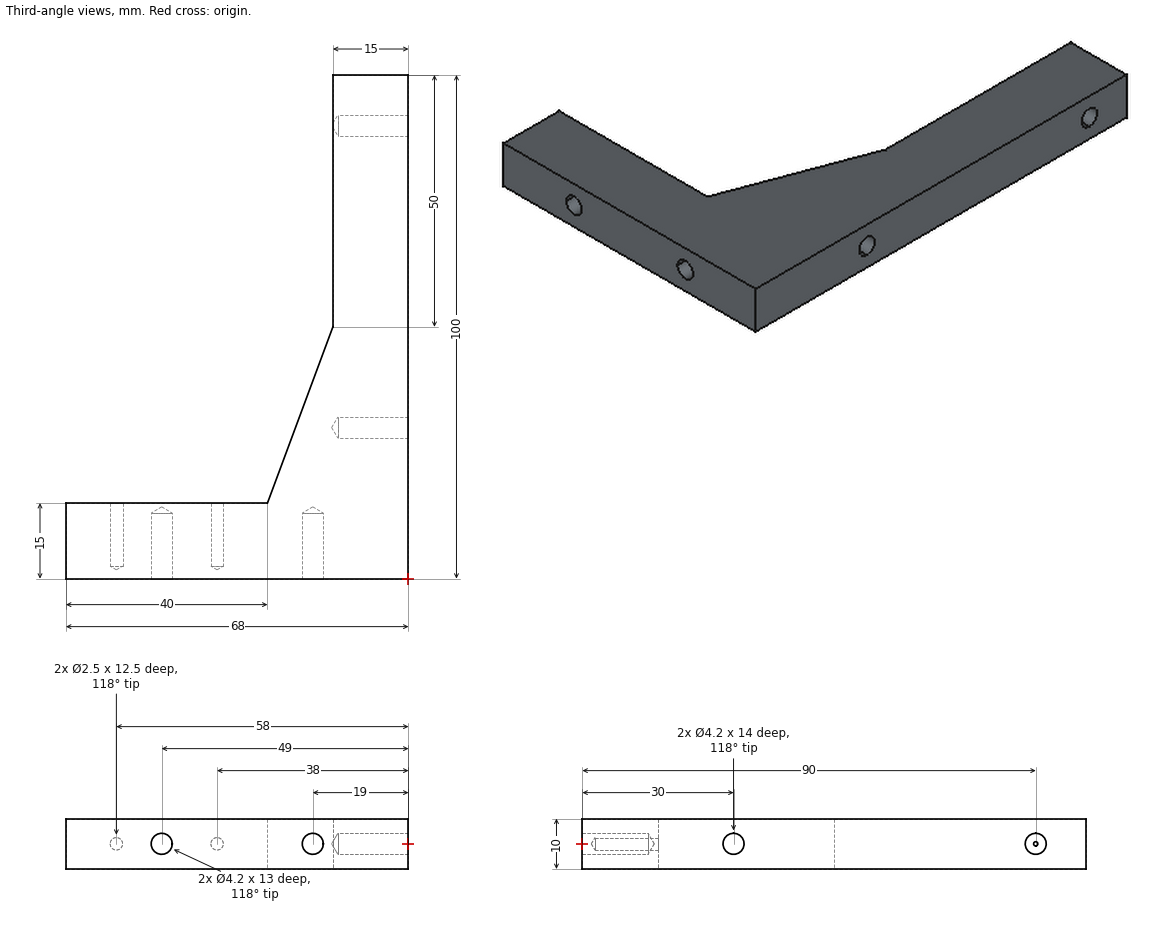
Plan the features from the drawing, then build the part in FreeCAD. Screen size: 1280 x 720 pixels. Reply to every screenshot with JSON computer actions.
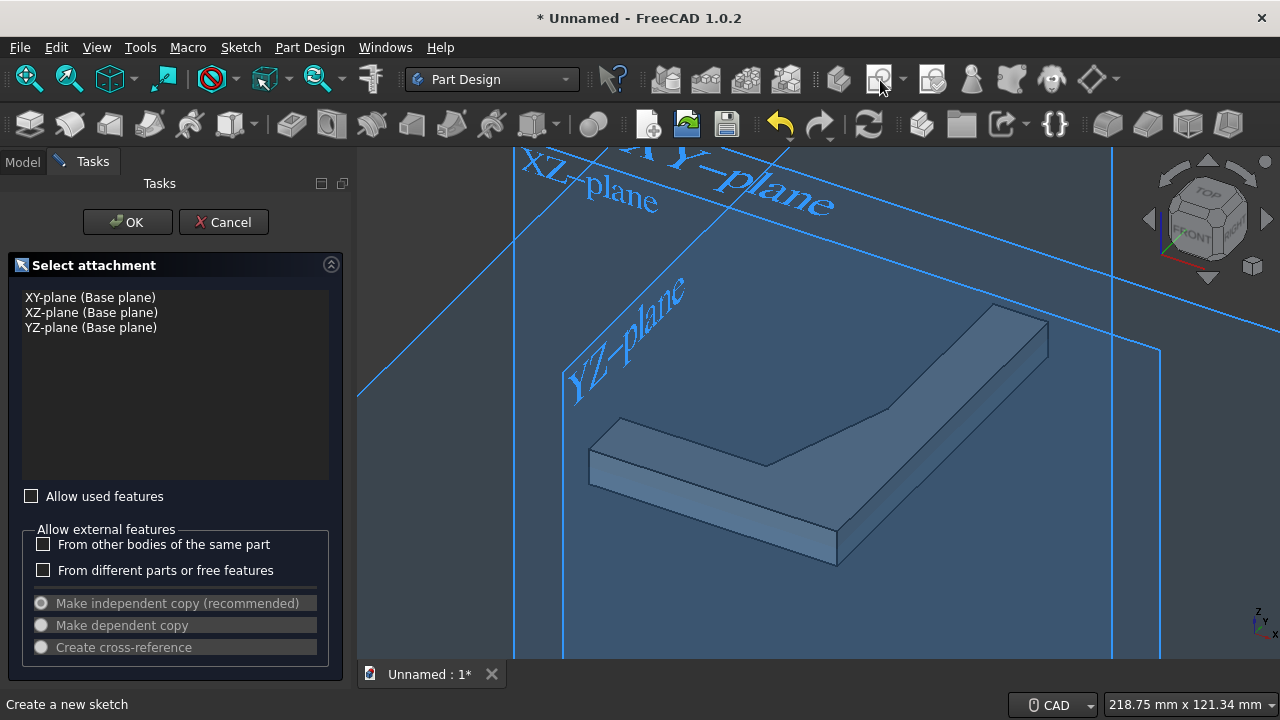
{"action": "left_click", "coordinate": [82, 312]}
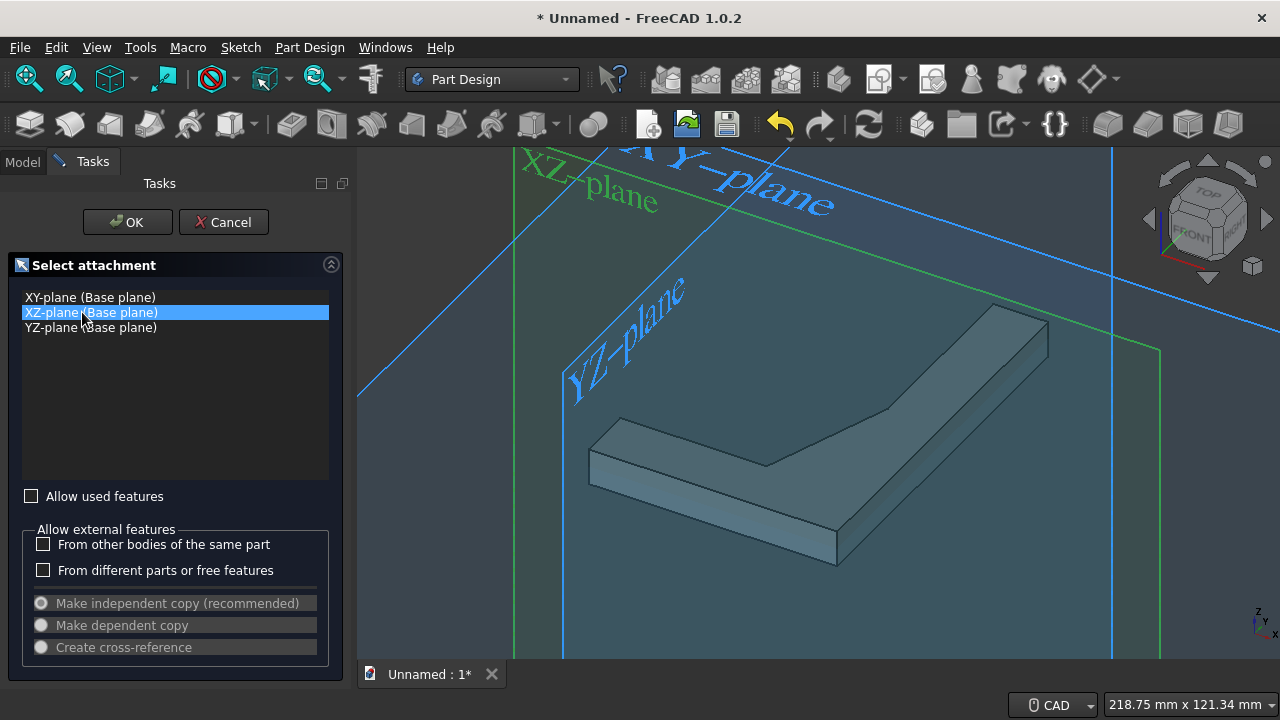
{"action": "left_click", "coordinate": [128, 222]}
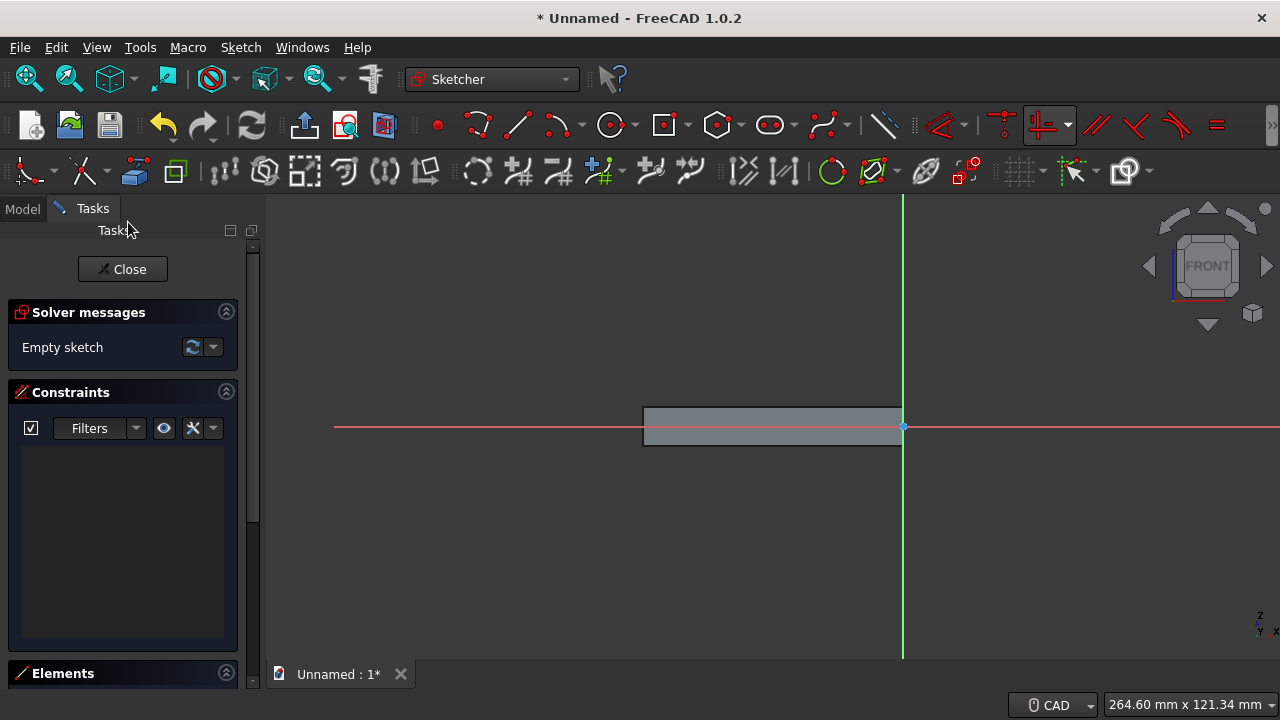
{"action": "scroll", "coordinate": [864, 427], "scroll_direction": "up", "scroll_amount": 5}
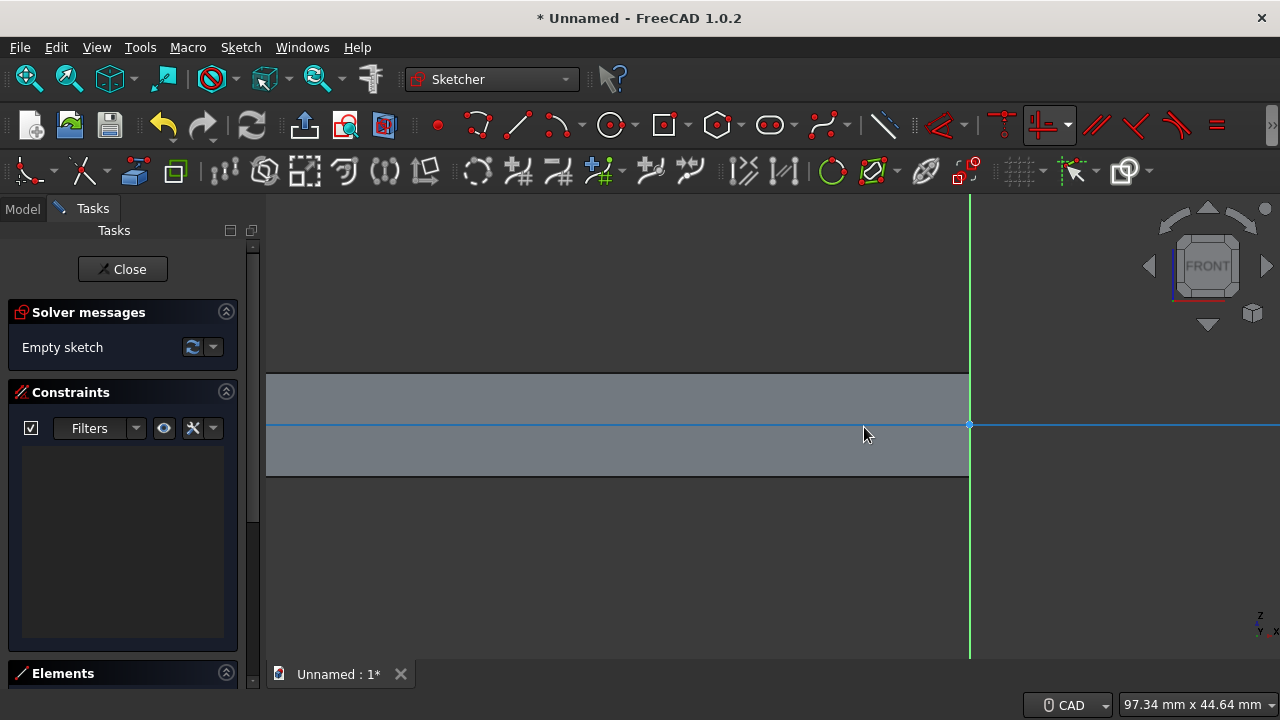
{"action": "key", "text": "g c"}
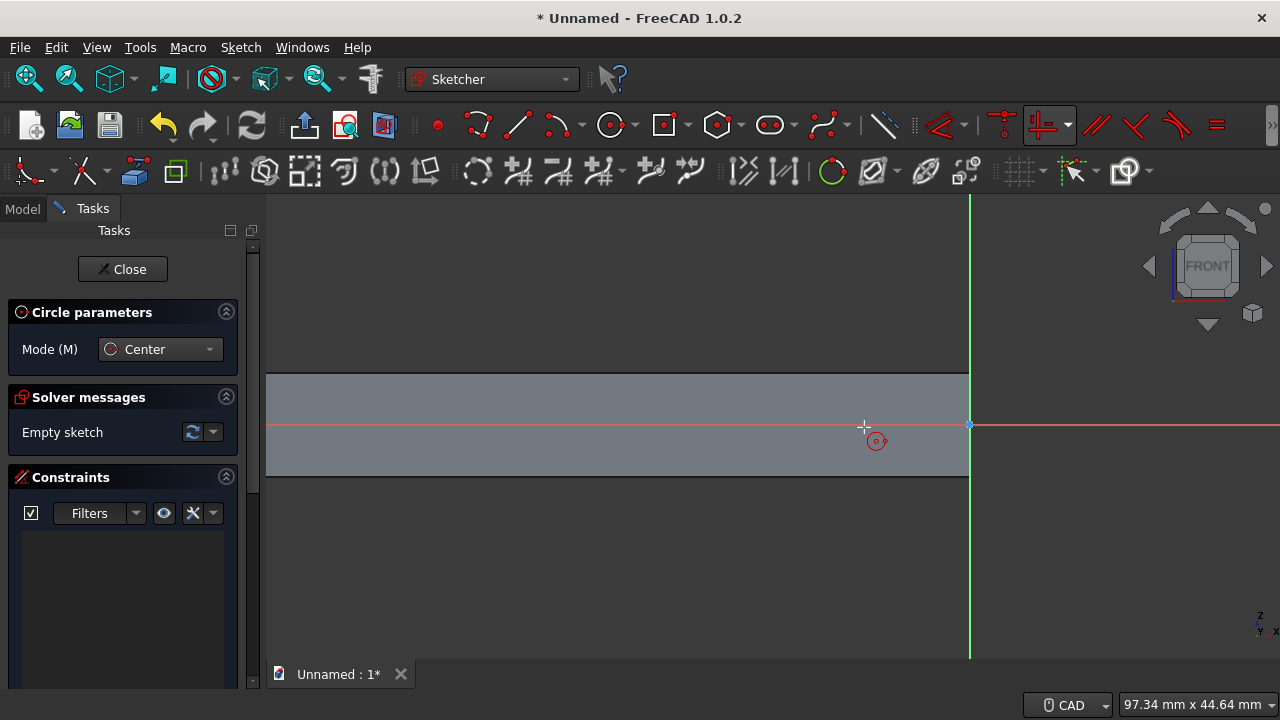
{"action": "left_click", "coordinate": [459, 425]}
{"action": "mouse_move", "coordinate": [475, 409]}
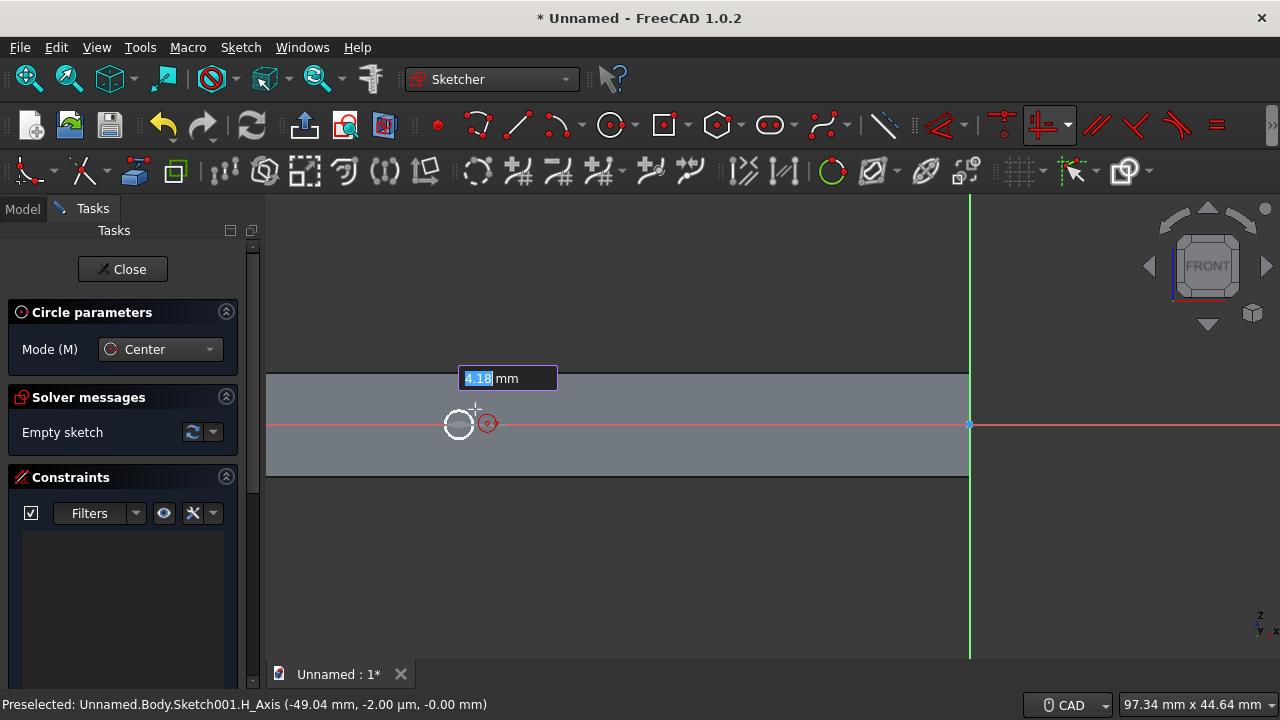
{"action": "type", "text": "4.2"}
{"action": "key", "text": "Return"}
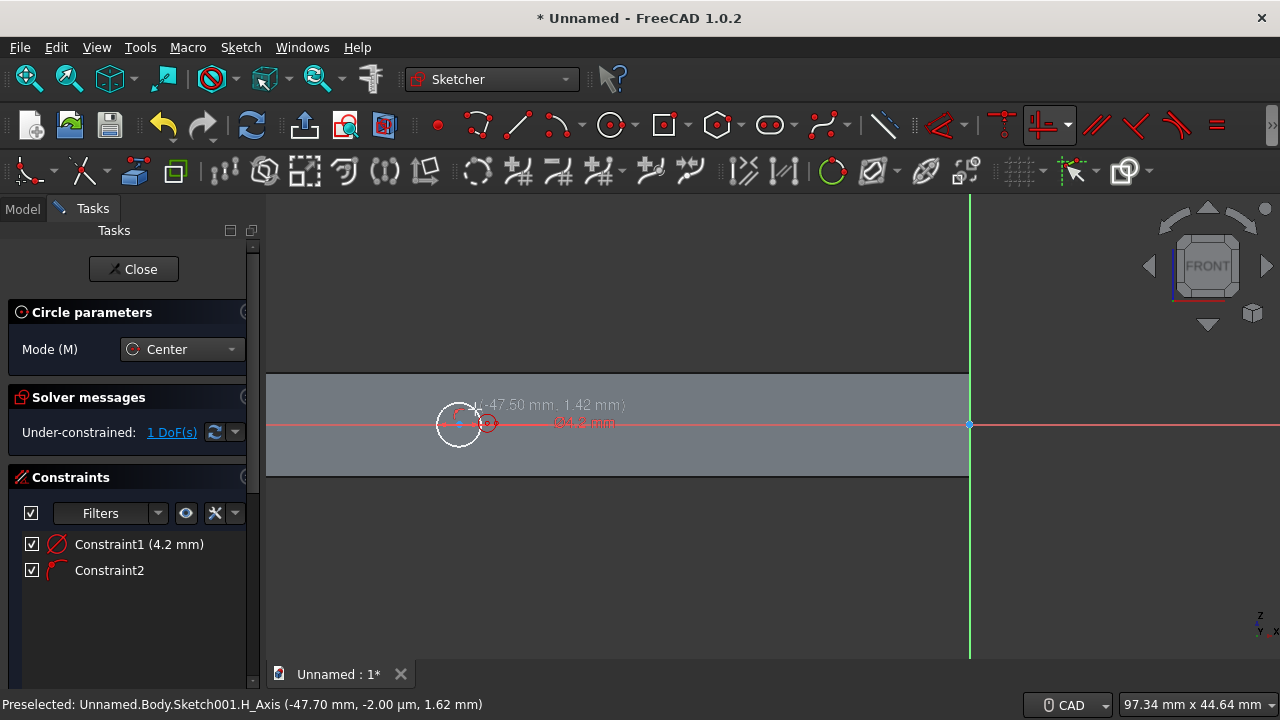
{"action": "left_click", "coordinate": [772, 425]}
{"action": "mouse_move", "coordinate": [787, 409]}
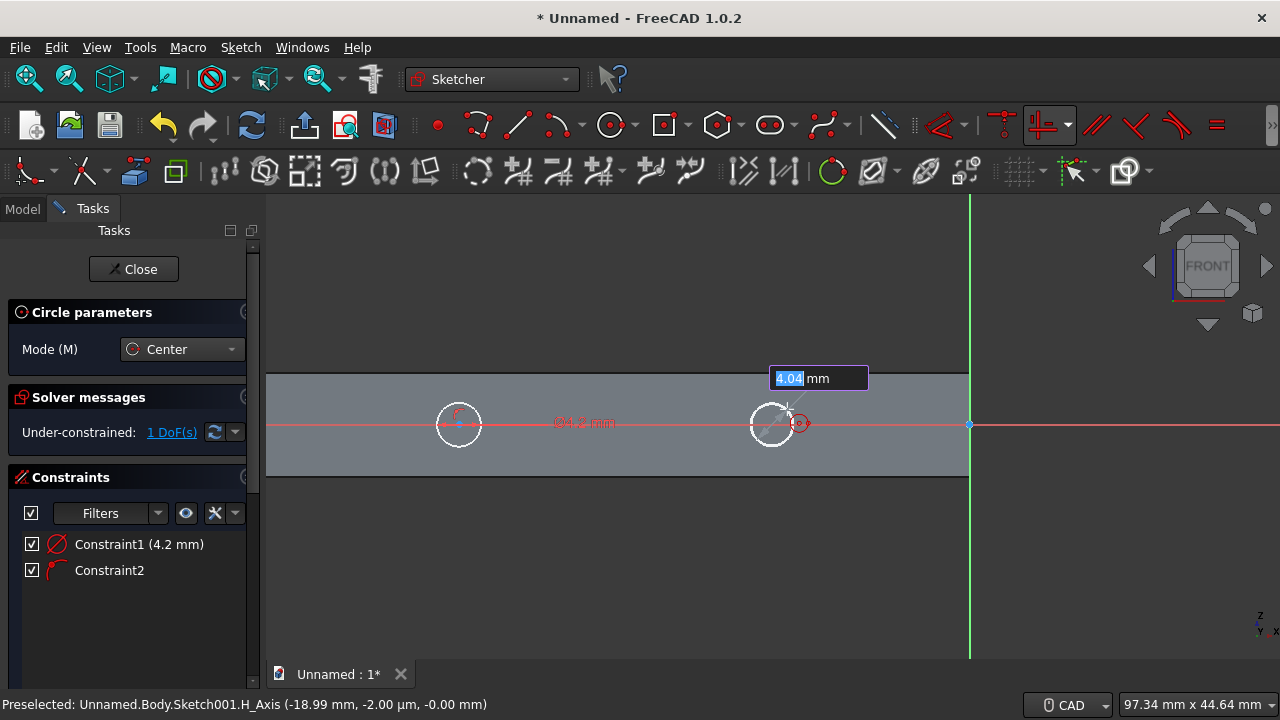
{"action": "type", "text": "4.2"}
{"action": "key", "text": "Return"}
{"action": "key", "text": "Escape"}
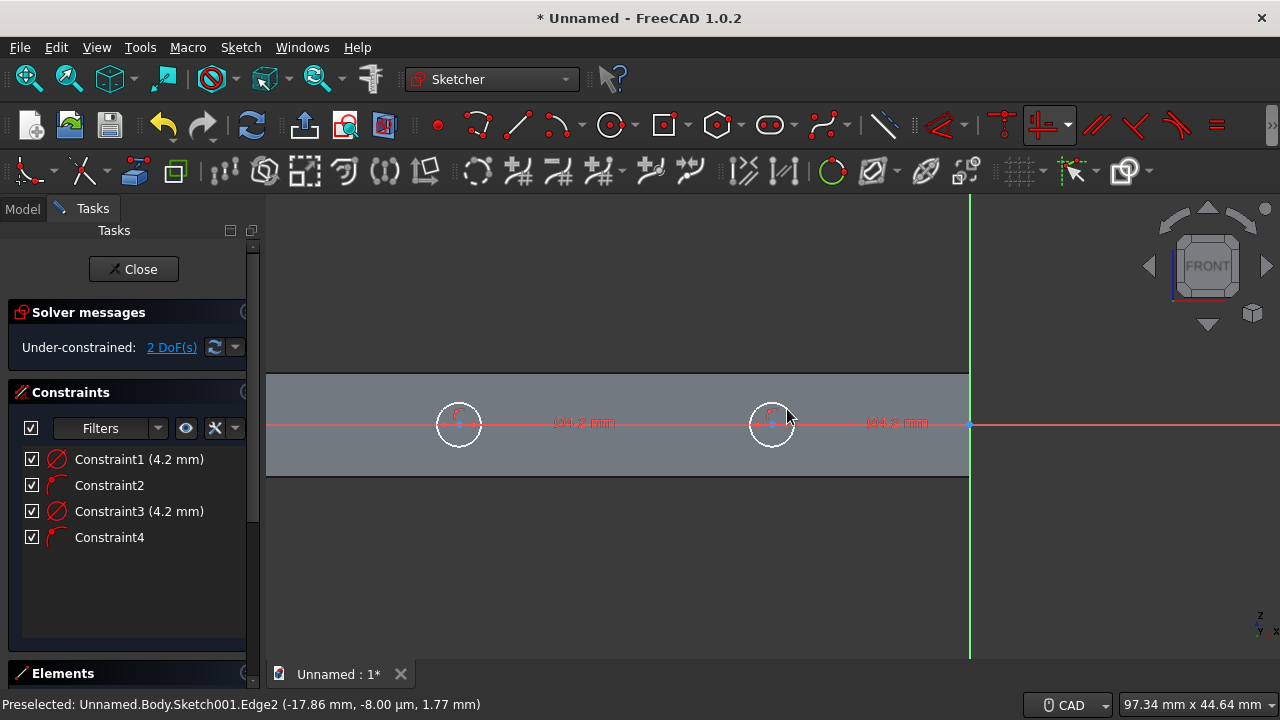
{"action": "key", "text": "d"}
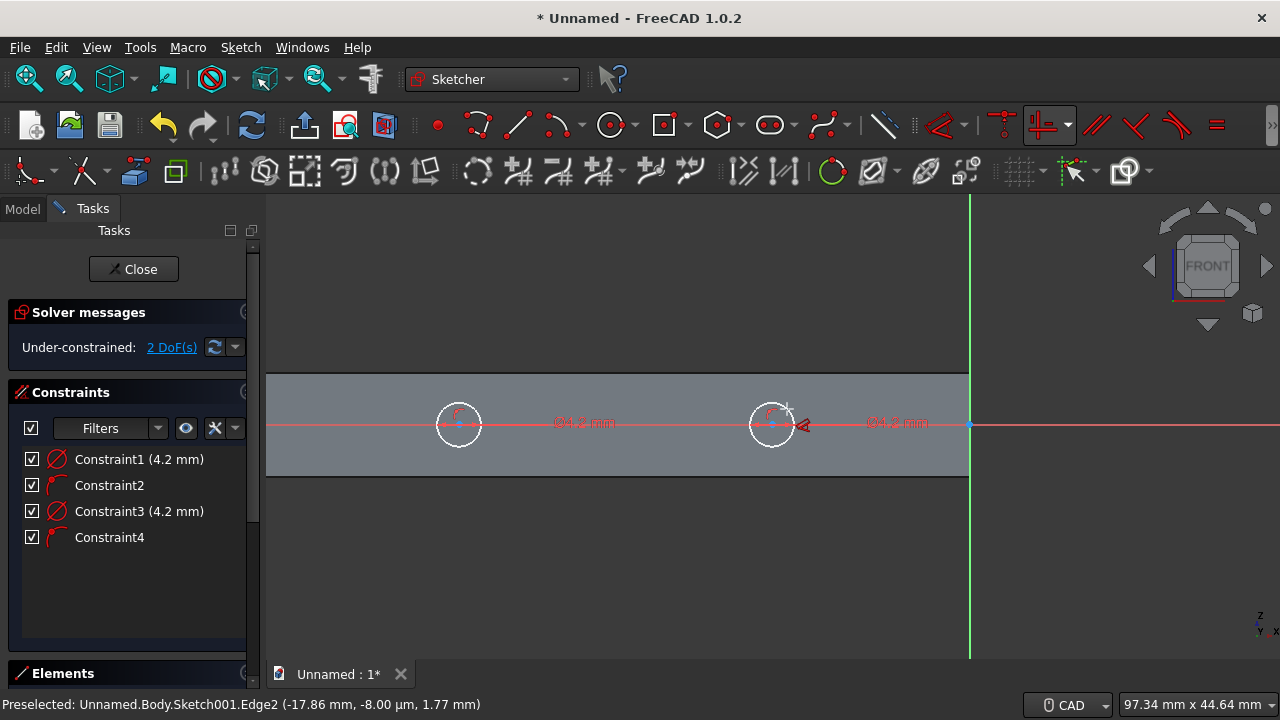
{"action": "left_click", "coordinate": [459, 425]}
{"action": "left_click", "coordinate": [714, 459]}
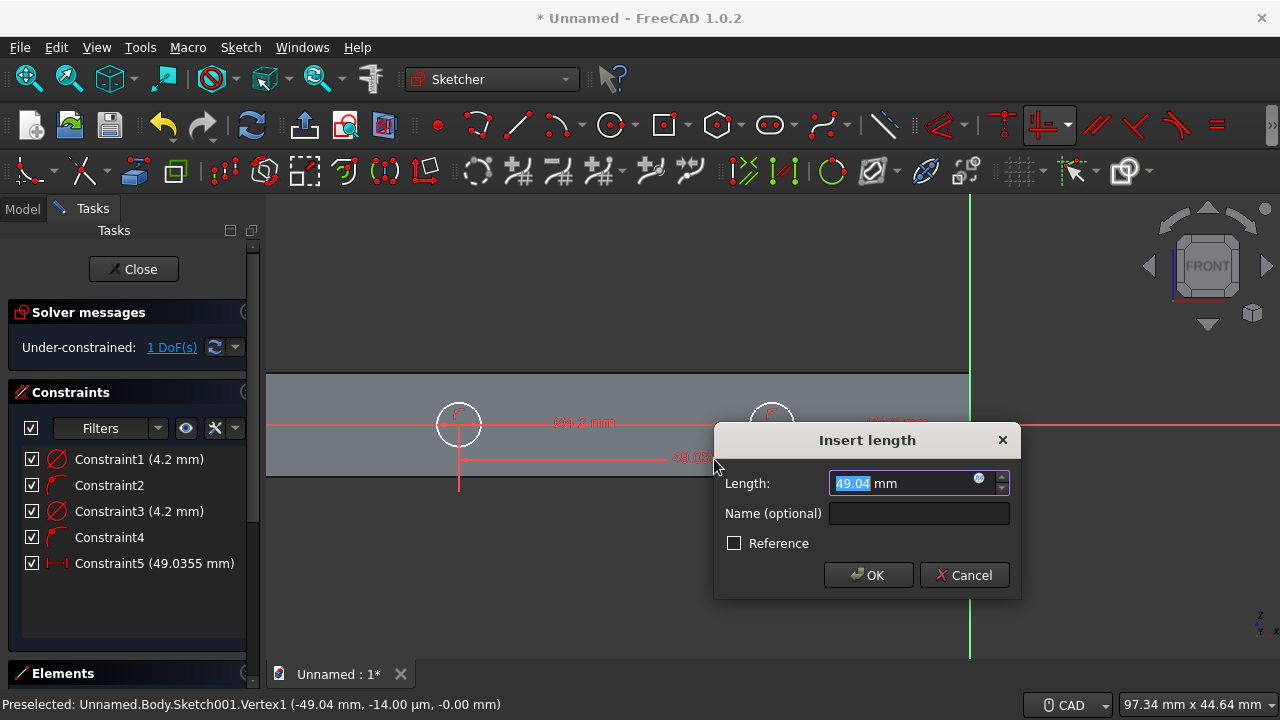
{"action": "type", "text": "49"}
{"action": "key", "text": "Return"}